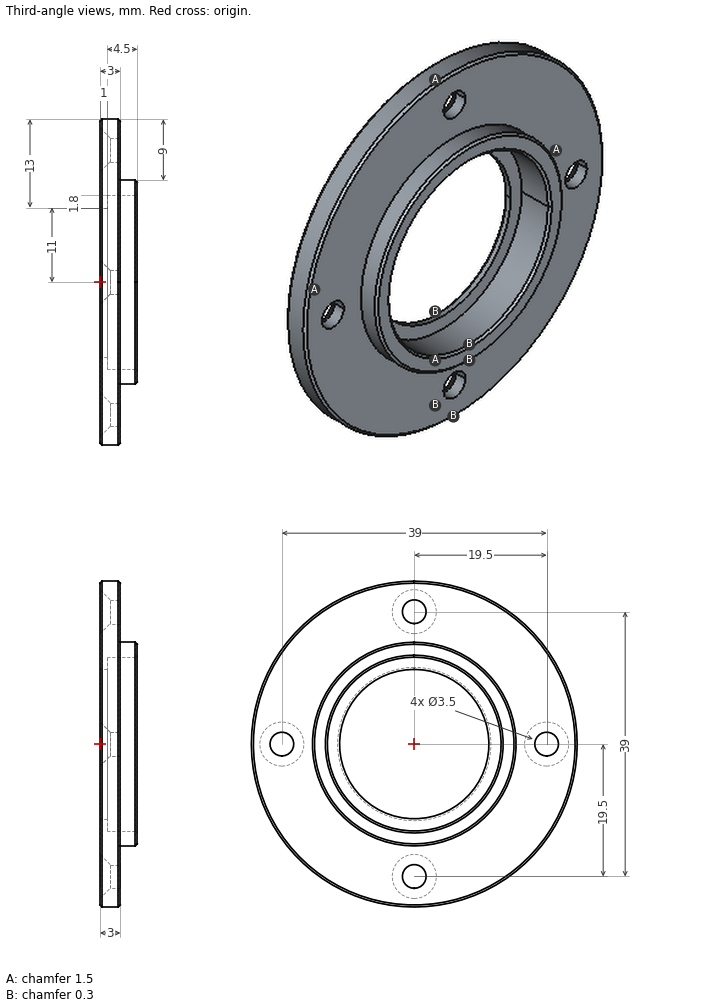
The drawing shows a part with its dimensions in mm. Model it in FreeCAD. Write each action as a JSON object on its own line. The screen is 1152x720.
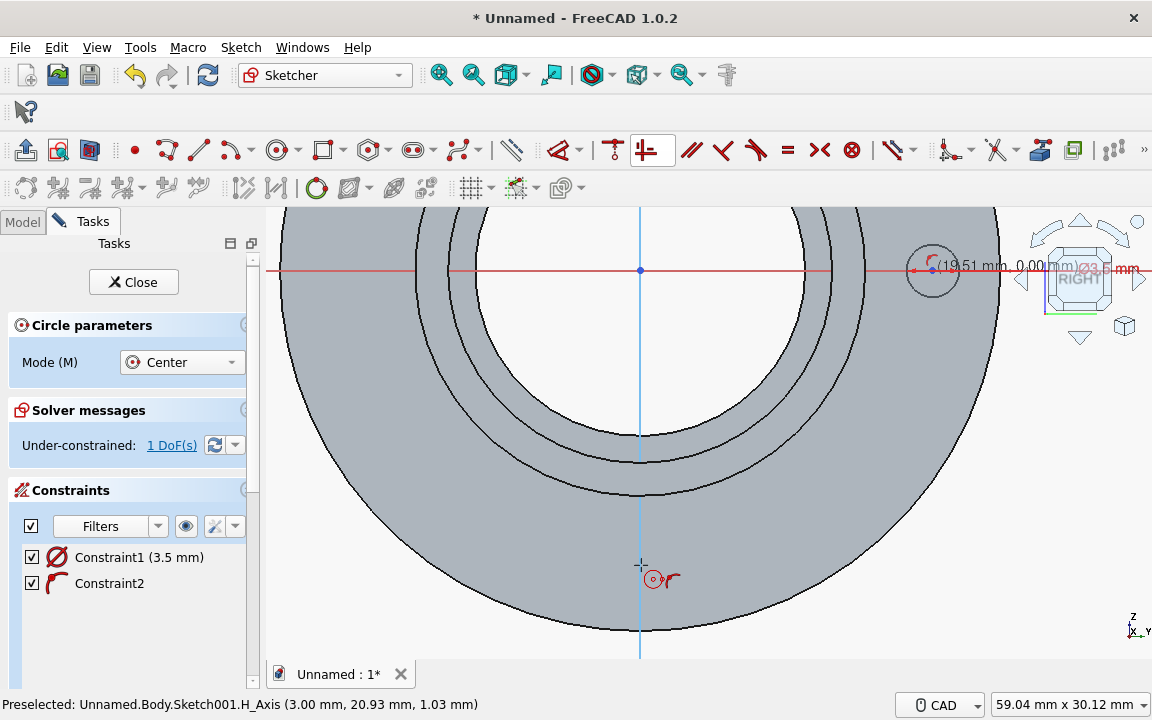
{"action": "left_click", "coordinate": [640, 564]}
{"action": "mouse_move", "coordinate": [659, 545]}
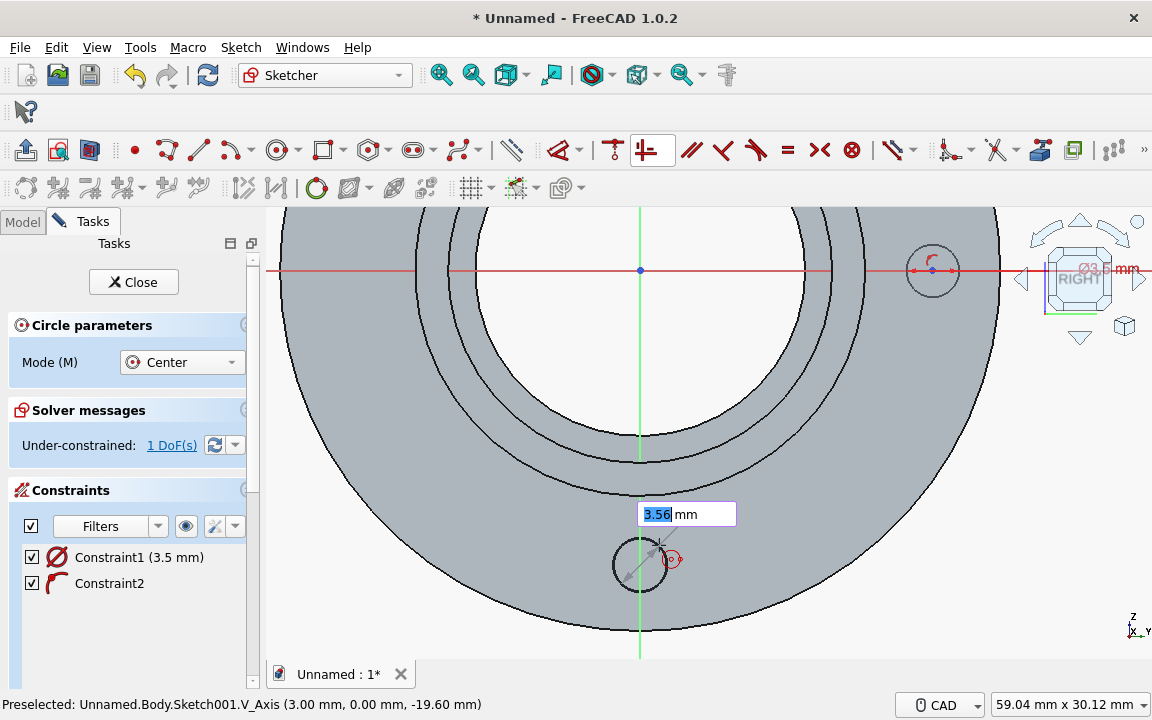
{"action": "type", "text": "3.5"}
{"action": "key", "text": "Return"}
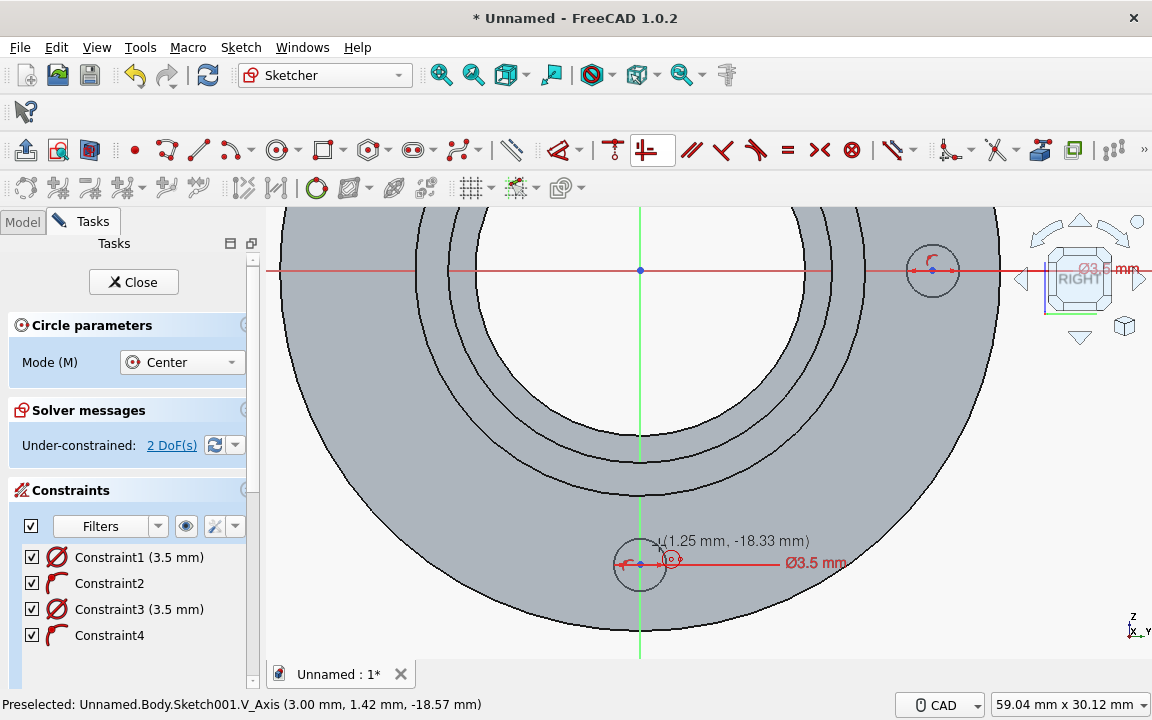
{"action": "left_click", "coordinate": [348, 271]}
{"action": "mouse_move", "coordinate": [366, 252]}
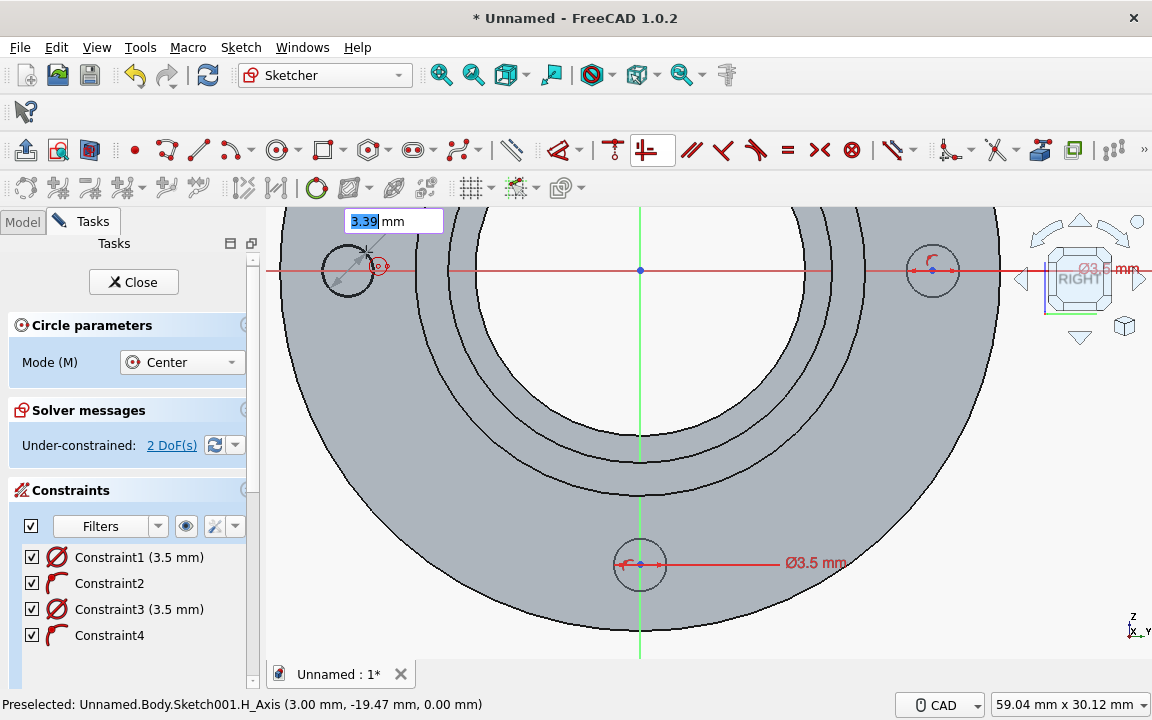
{"action": "type", "text": "3.5"}
{"action": "key", "text": "Return"}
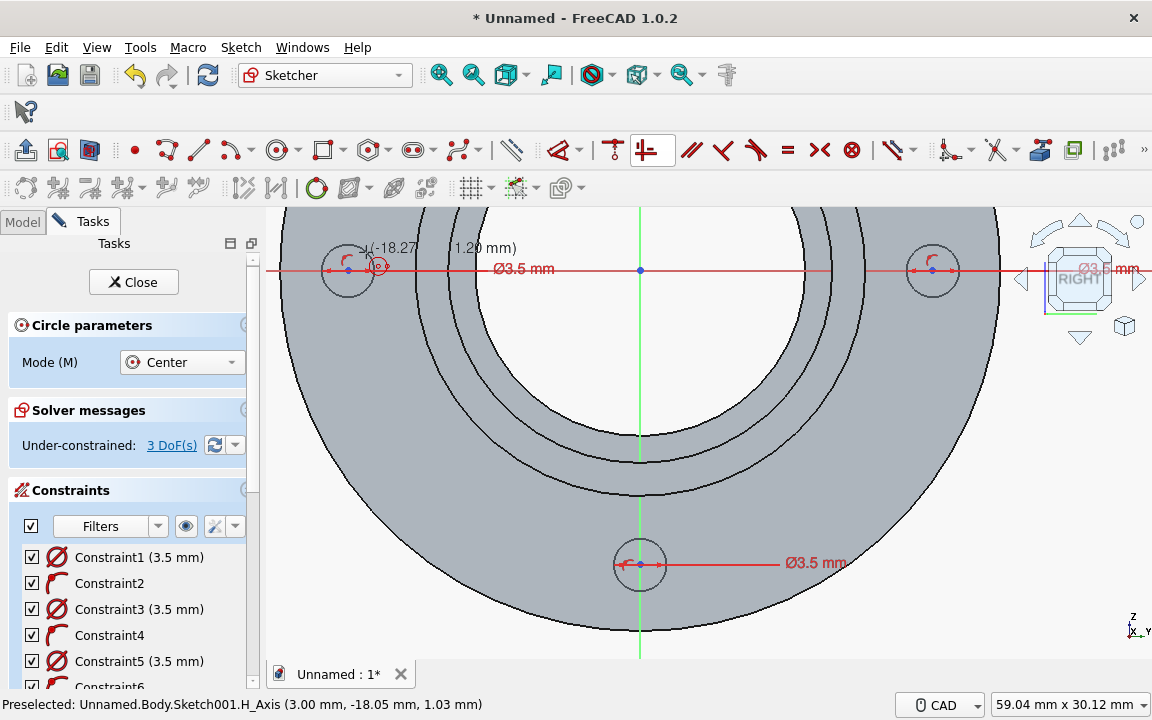
{"action": "scroll", "coordinate": [641, 565], "scroll_direction": "down", "scroll_amount": 4}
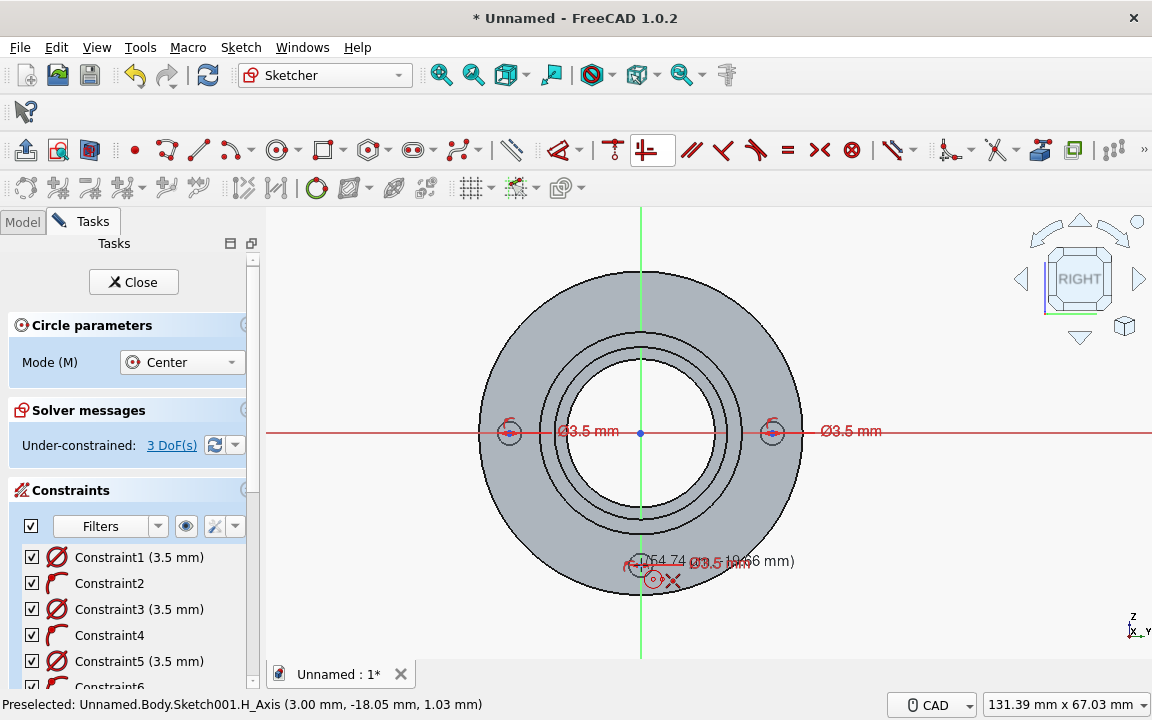
{"action": "scroll", "coordinate": [641, 302], "scroll_direction": "up", "scroll_amount": 4}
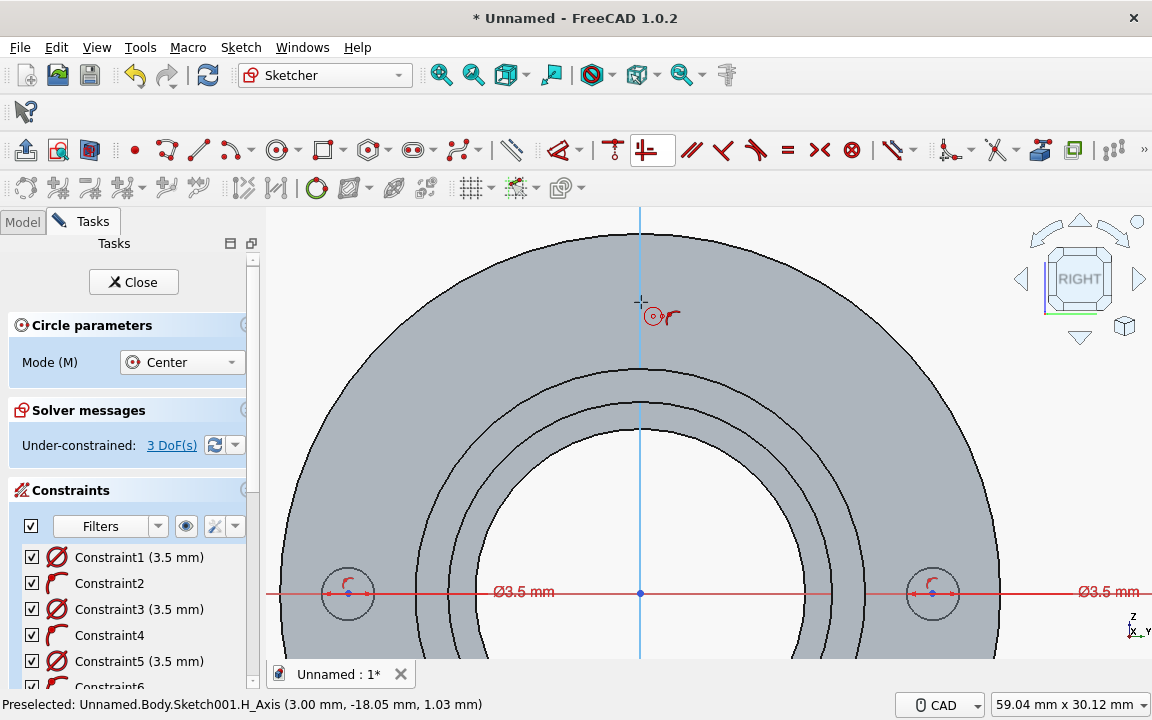
{"action": "left_click", "coordinate": [640, 301]}
{"action": "mouse_move", "coordinate": [659, 283]}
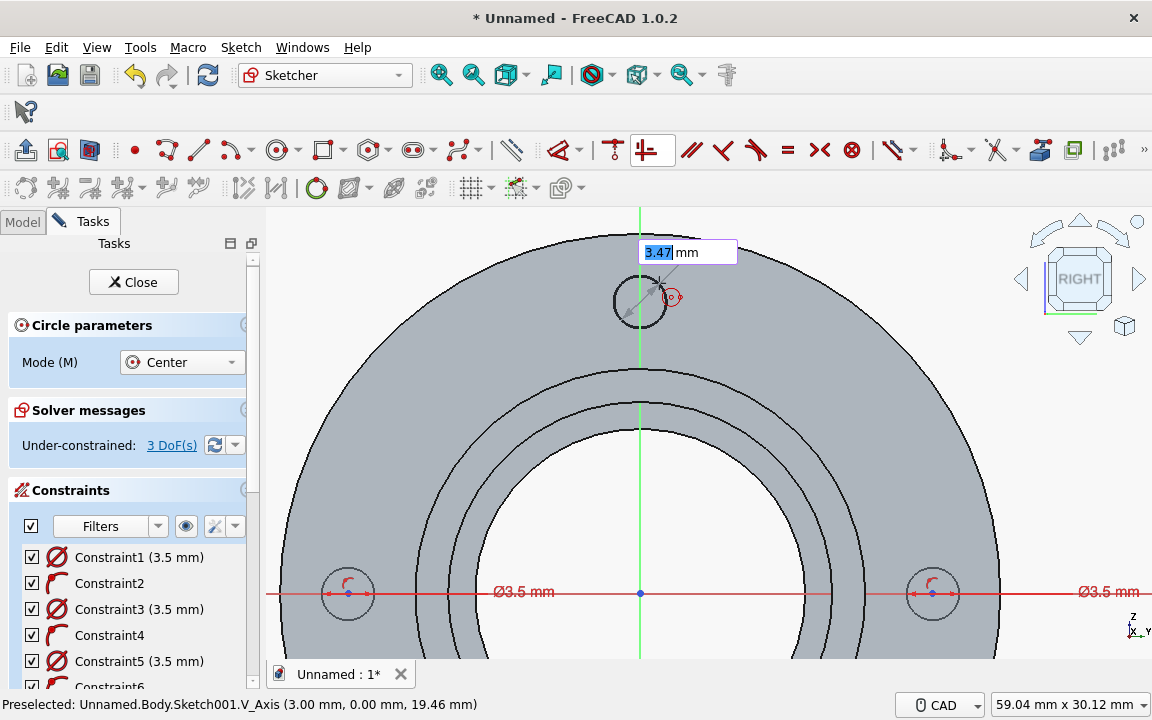
{"action": "type", "text": "3.5"}
{"action": "key", "text": "Return"}
{"action": "key", "text": "Escape"}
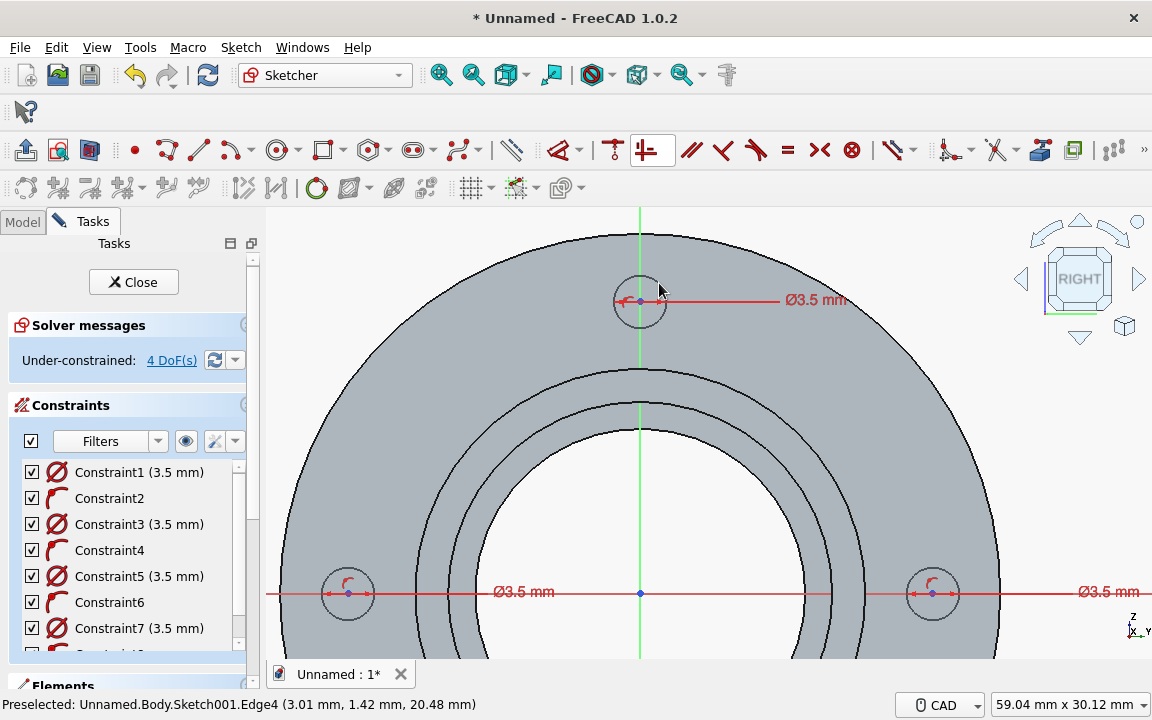
{"action": "left_click", "coordinate": [558, 150]}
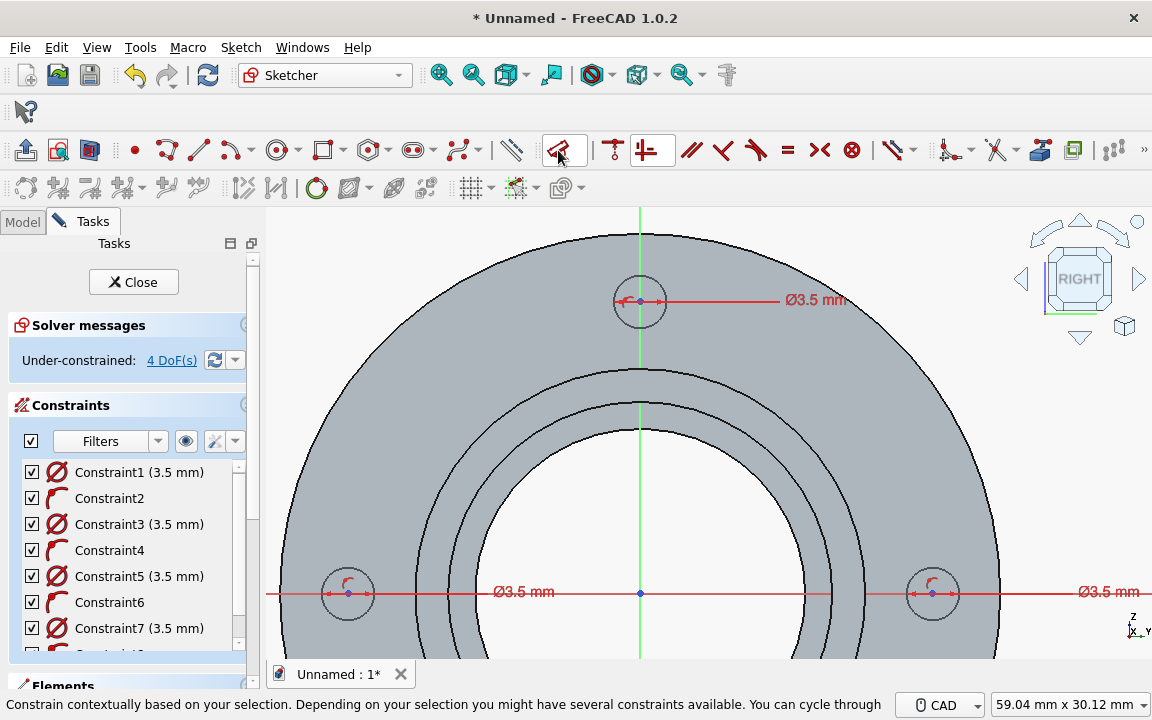
{"action": "left_click", "coordinate": [933, 594]}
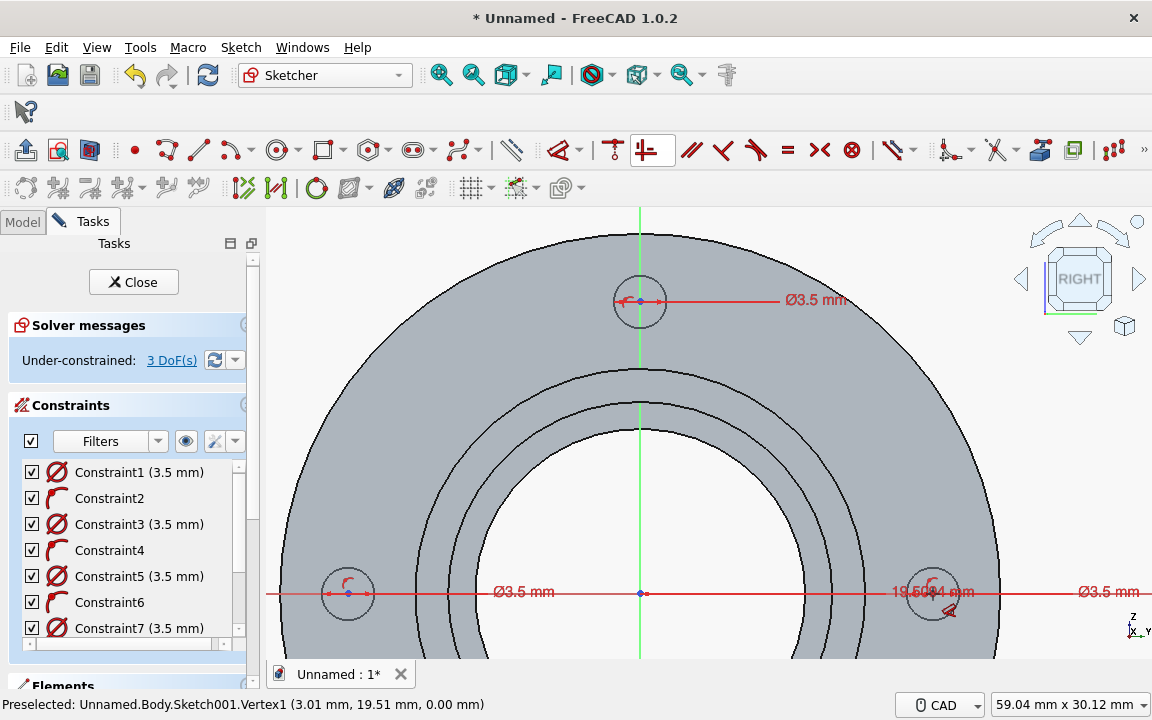
{"action": "left_click", "coordinate": [348, 594]}
{"action": "left_click", "coordinate": [506, 628]}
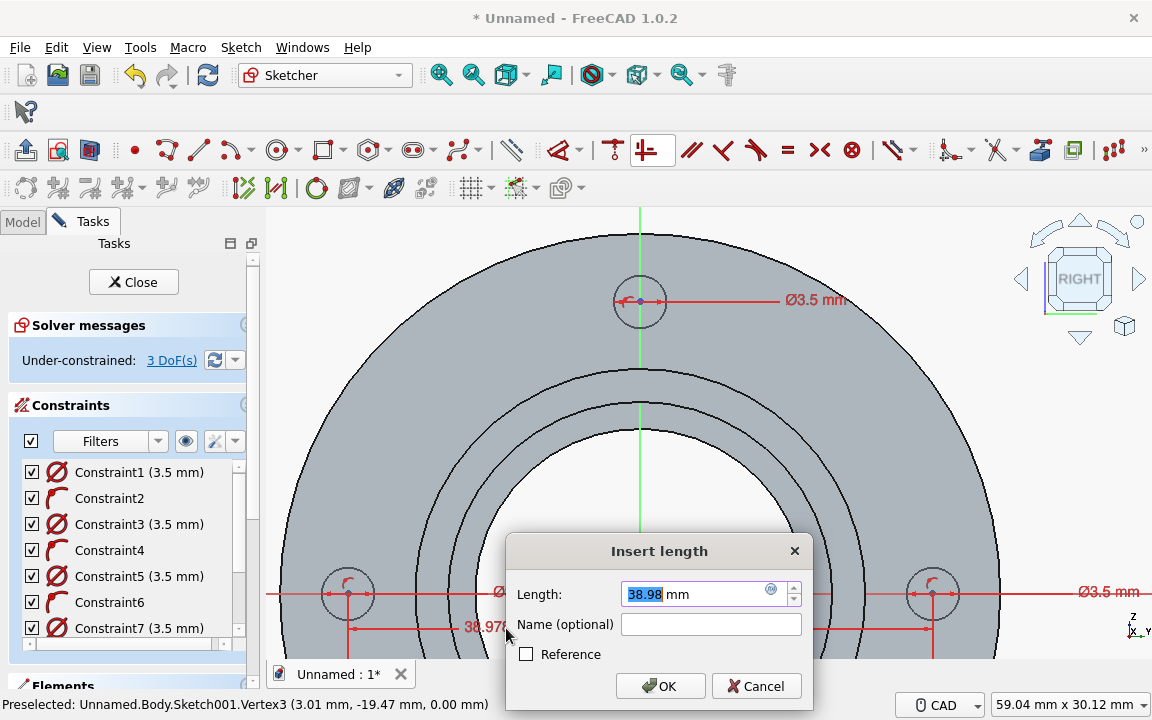
{"action": "type", "text": "39"}
{"action": "key", "text": "Return"}